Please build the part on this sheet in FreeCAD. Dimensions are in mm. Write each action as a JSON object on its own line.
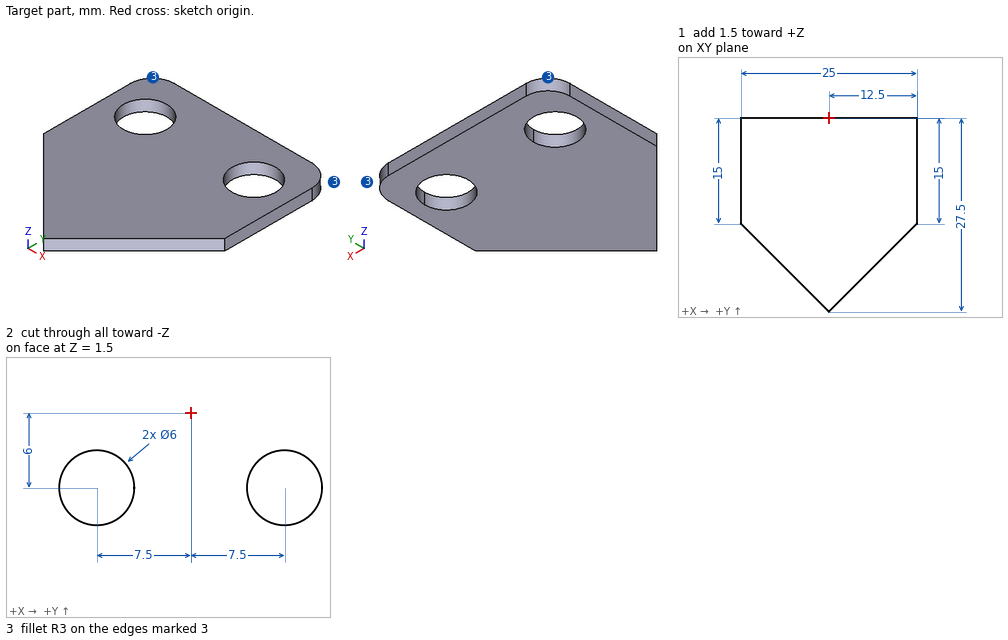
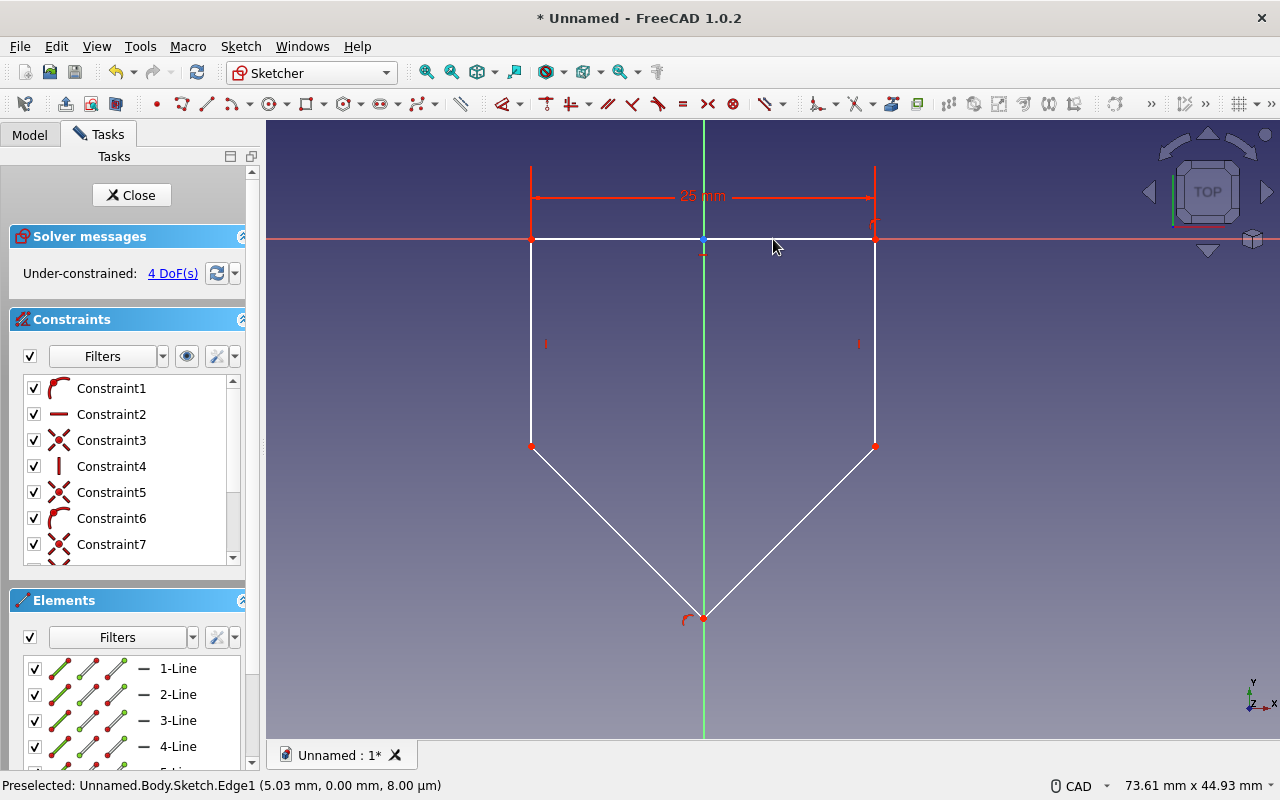
{"action": "left_click", "coordinate": [531, 302]}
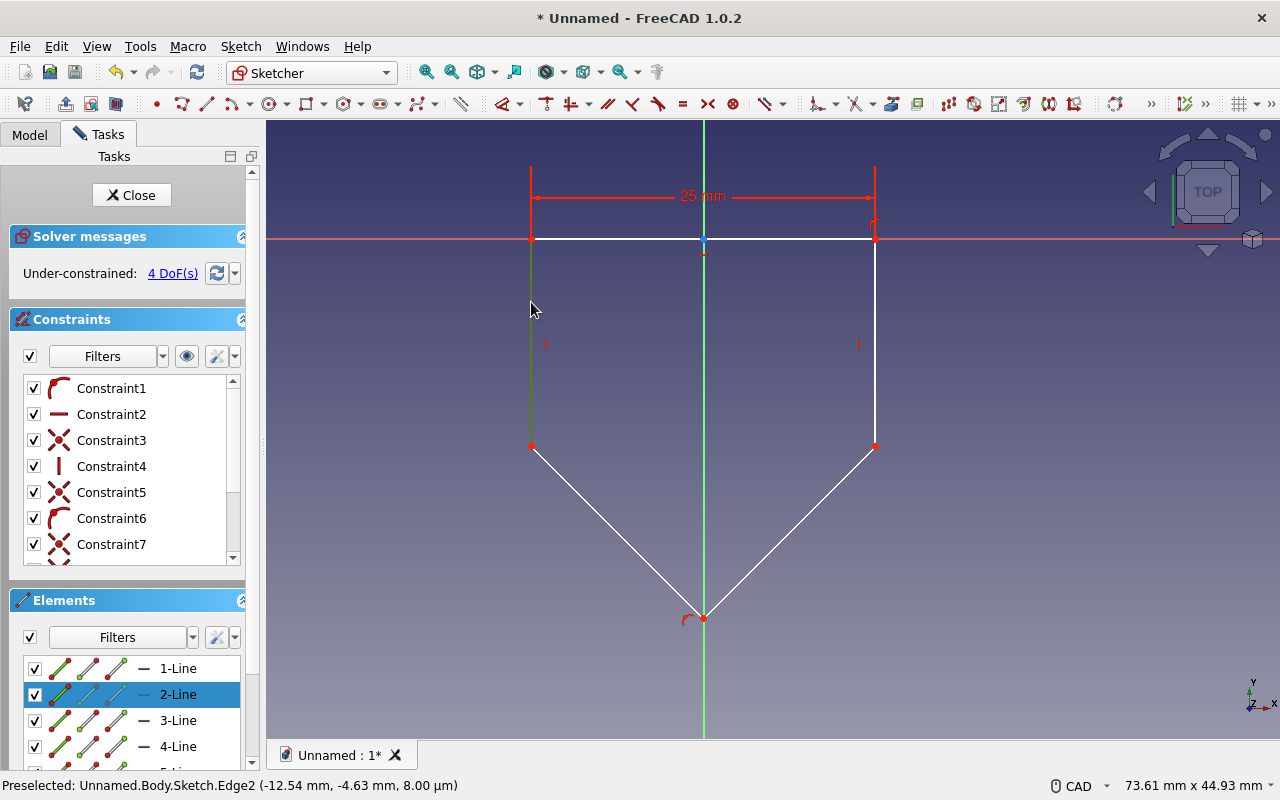
{"action": "left_click", "coordinate": [520, 104]}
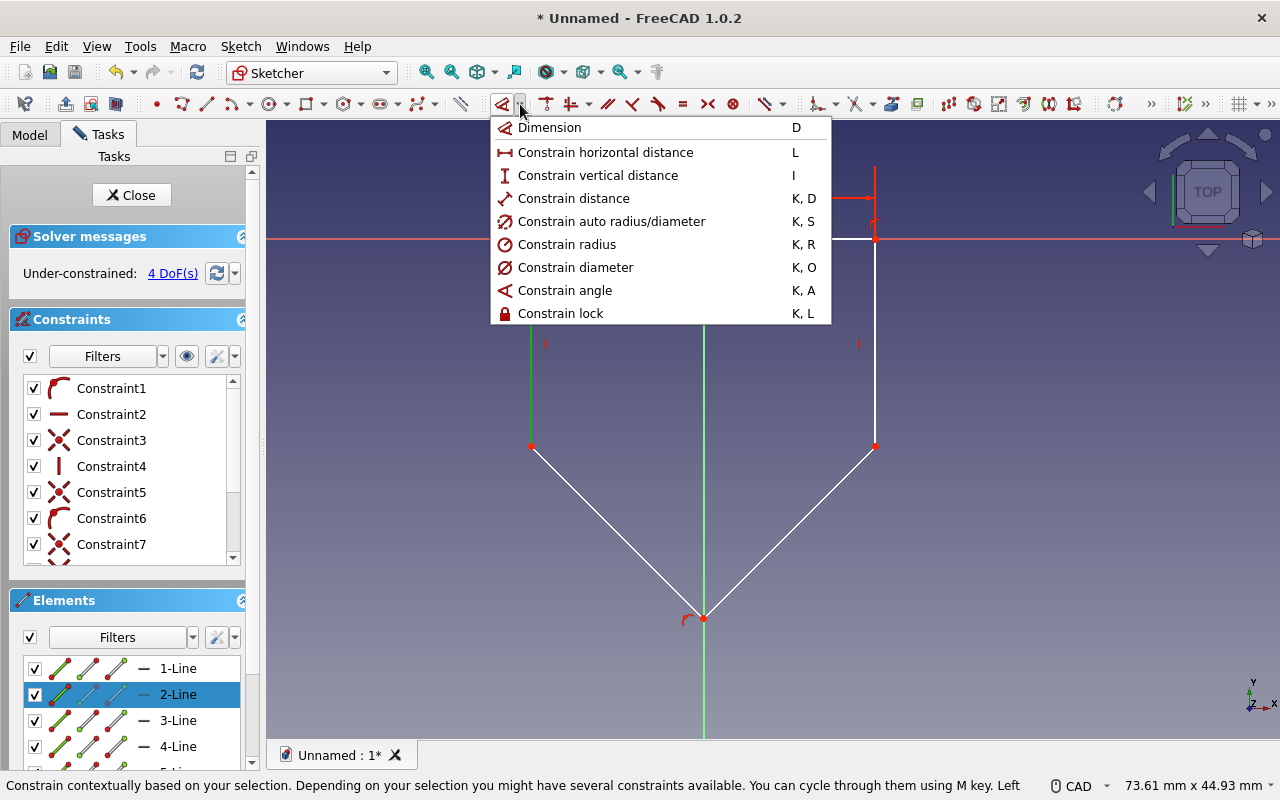
{"action": "left_click", "coordinate": [661, 176]}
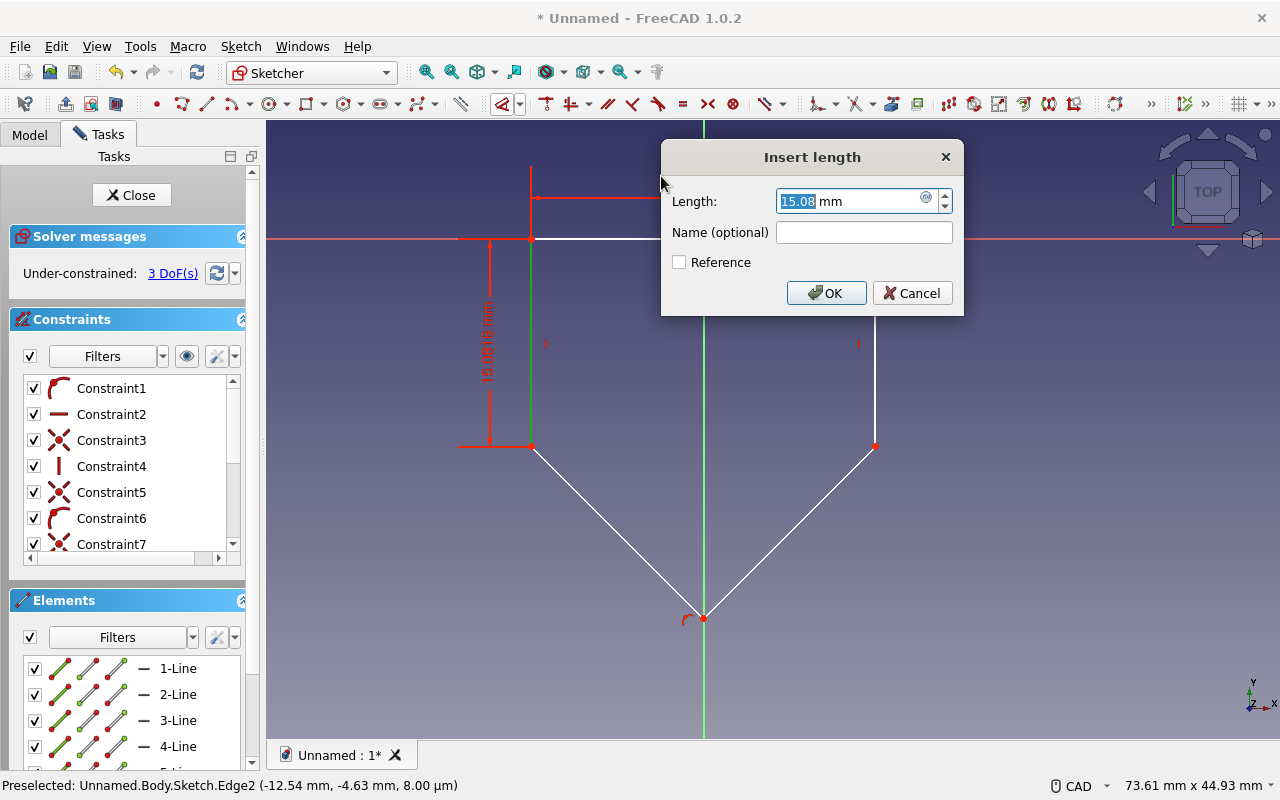
{"action": "type", "text": "15"}
{"action": "key", "text": "Return"}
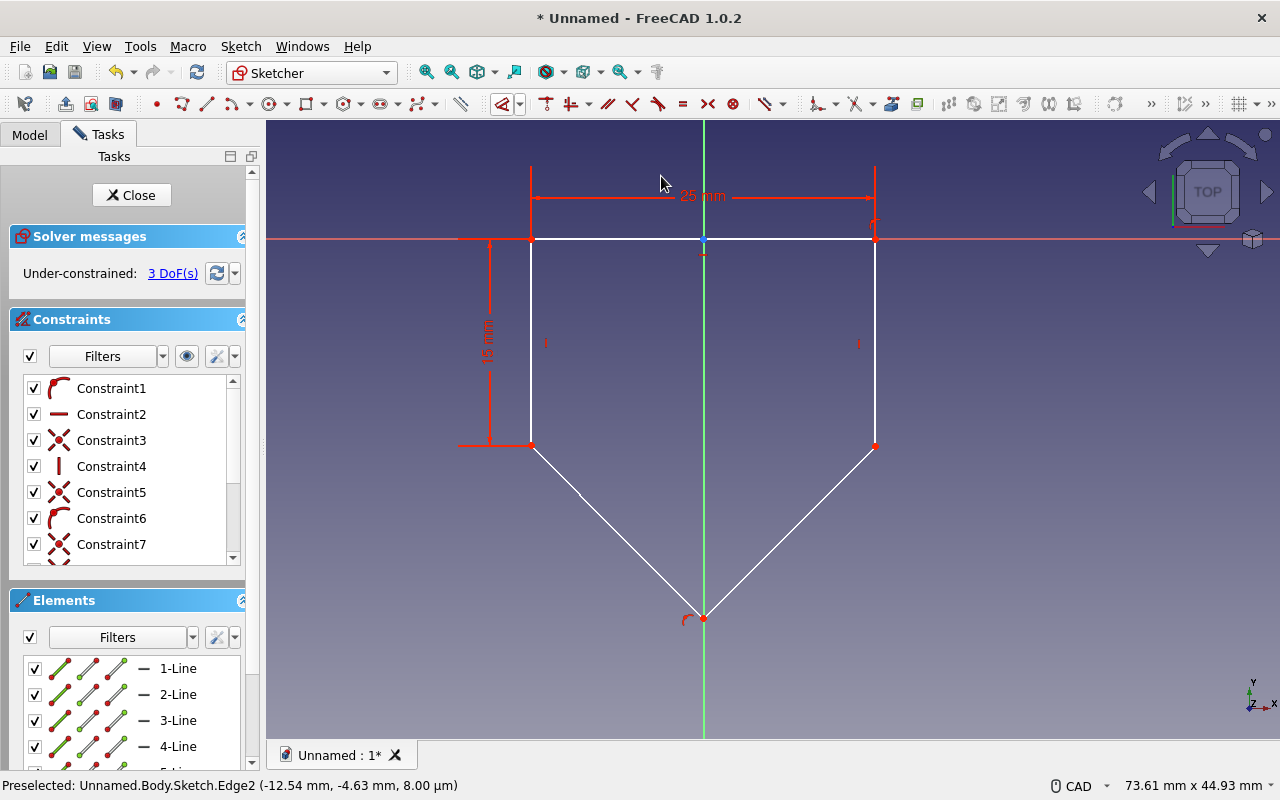
{"action": "left_click", "coordinate": [875, 385]}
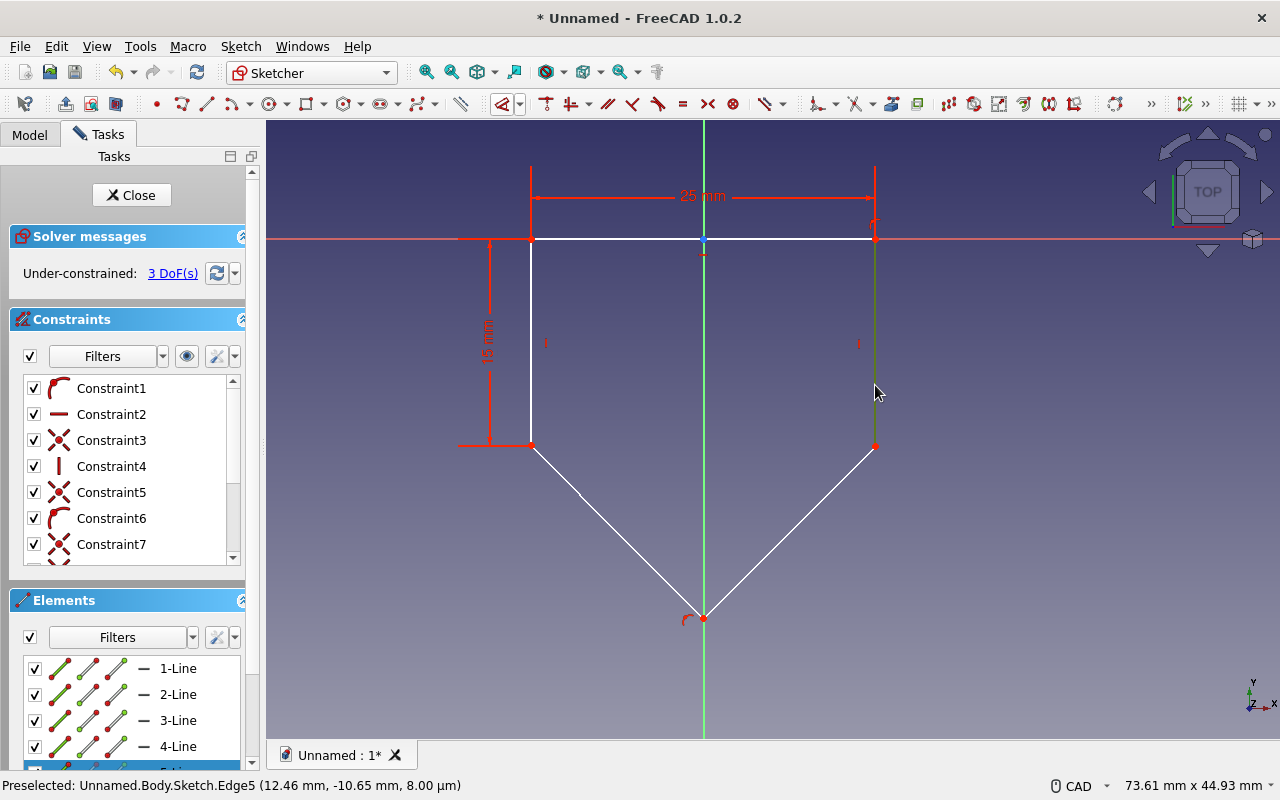
{"action": "left_click", "coordinate": [520, 104]}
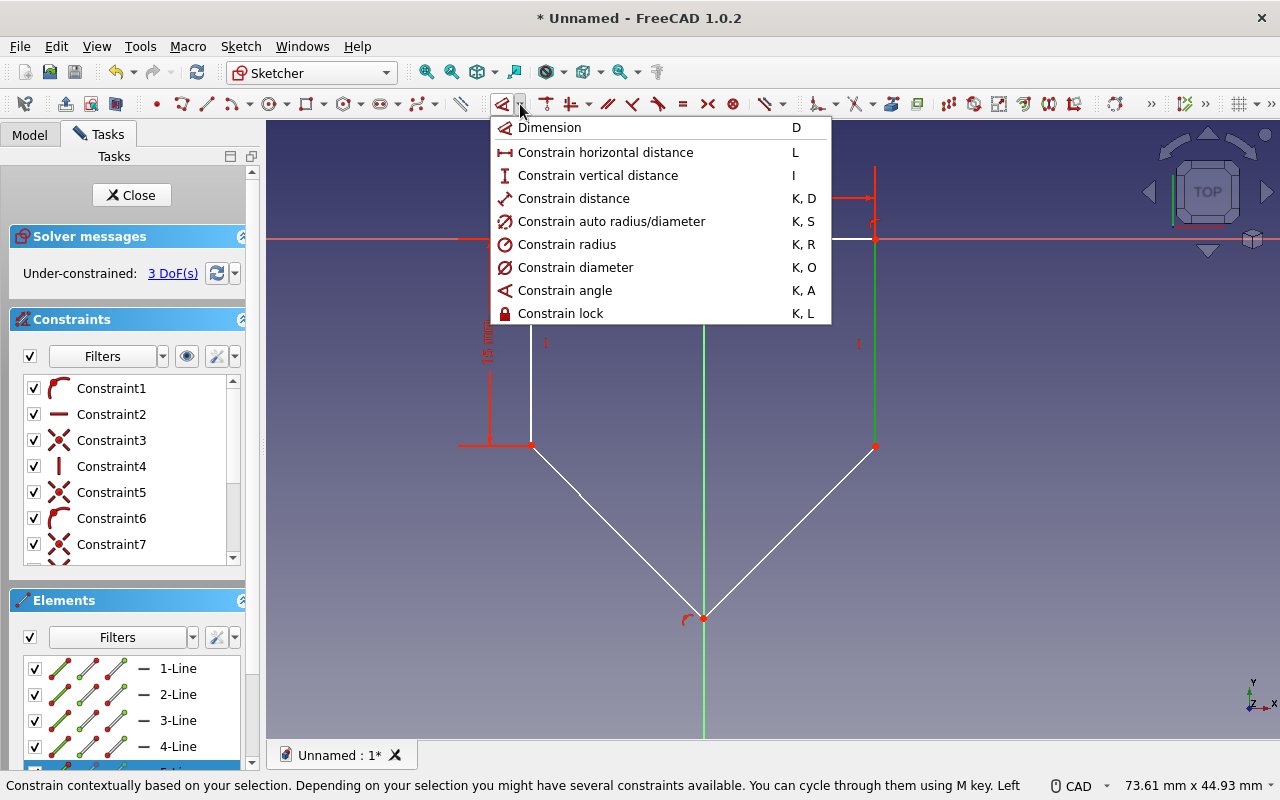
{"action": "left_click", "coordinate": [661, 176]}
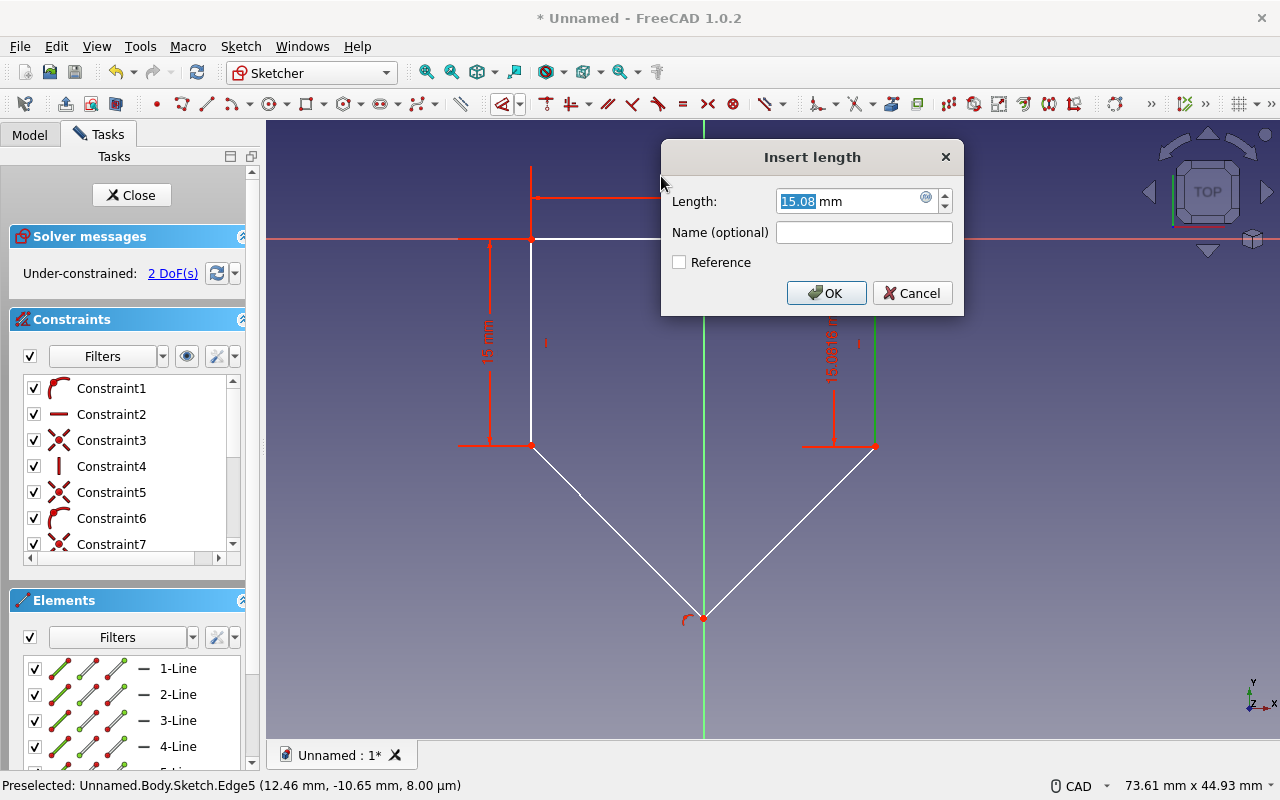
{"action": "type", "text": "15"}
{"action": "key", "text": "Return"}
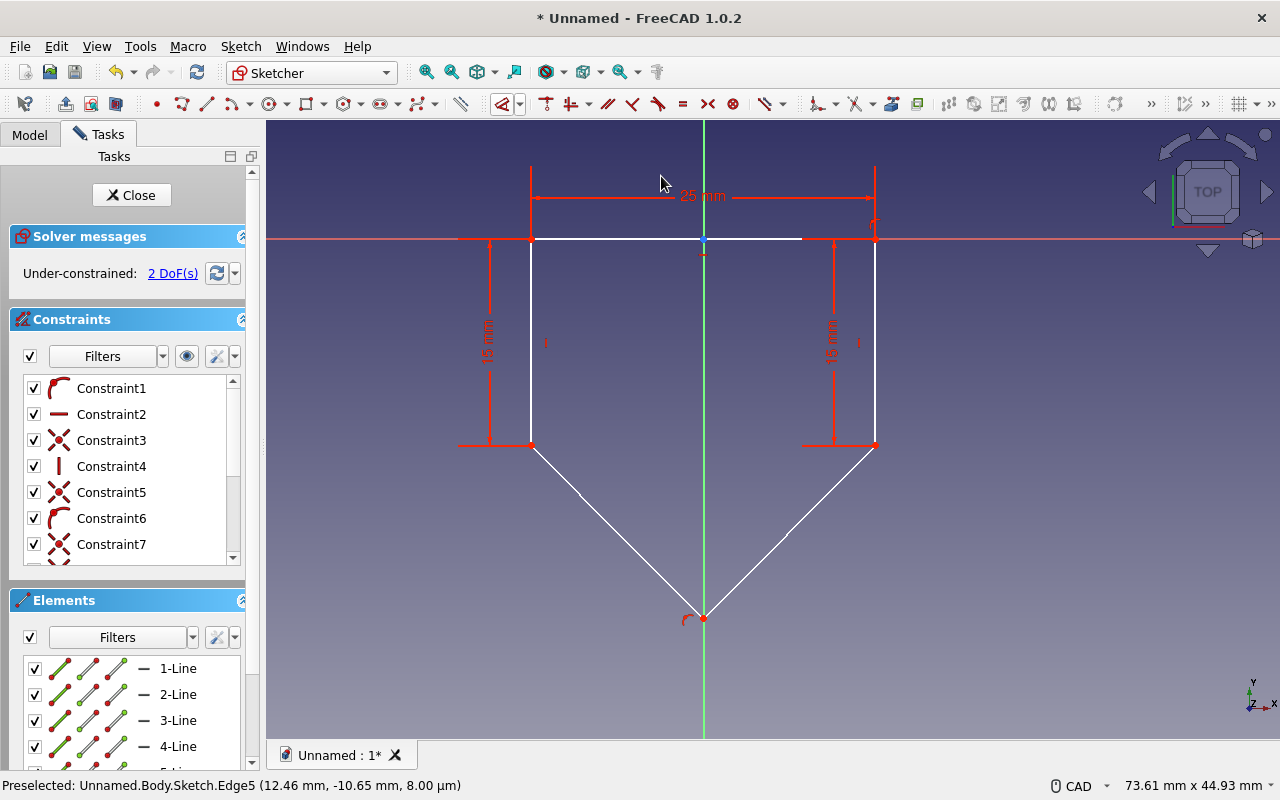
{"action": "left_click", "coordinate": [875, 239]}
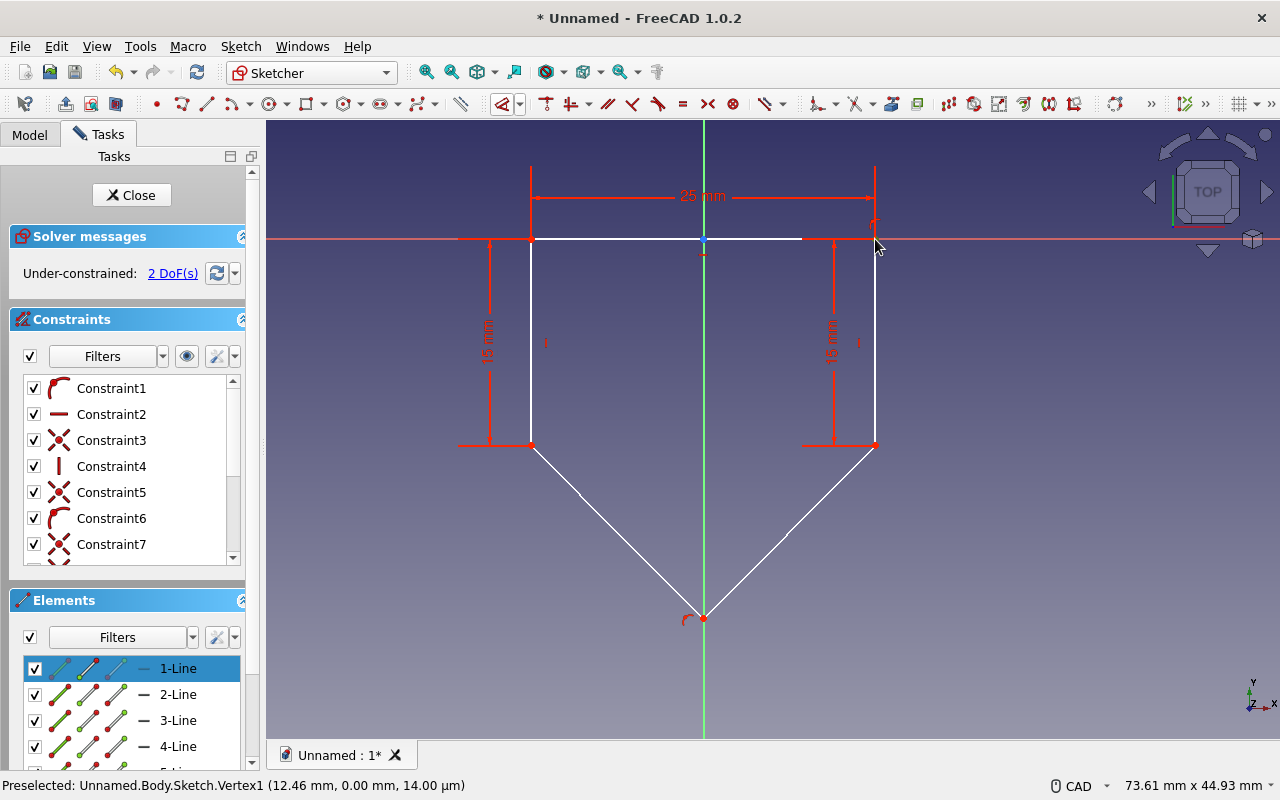
{"action": "left_click", "coordinate": [520, 104]}